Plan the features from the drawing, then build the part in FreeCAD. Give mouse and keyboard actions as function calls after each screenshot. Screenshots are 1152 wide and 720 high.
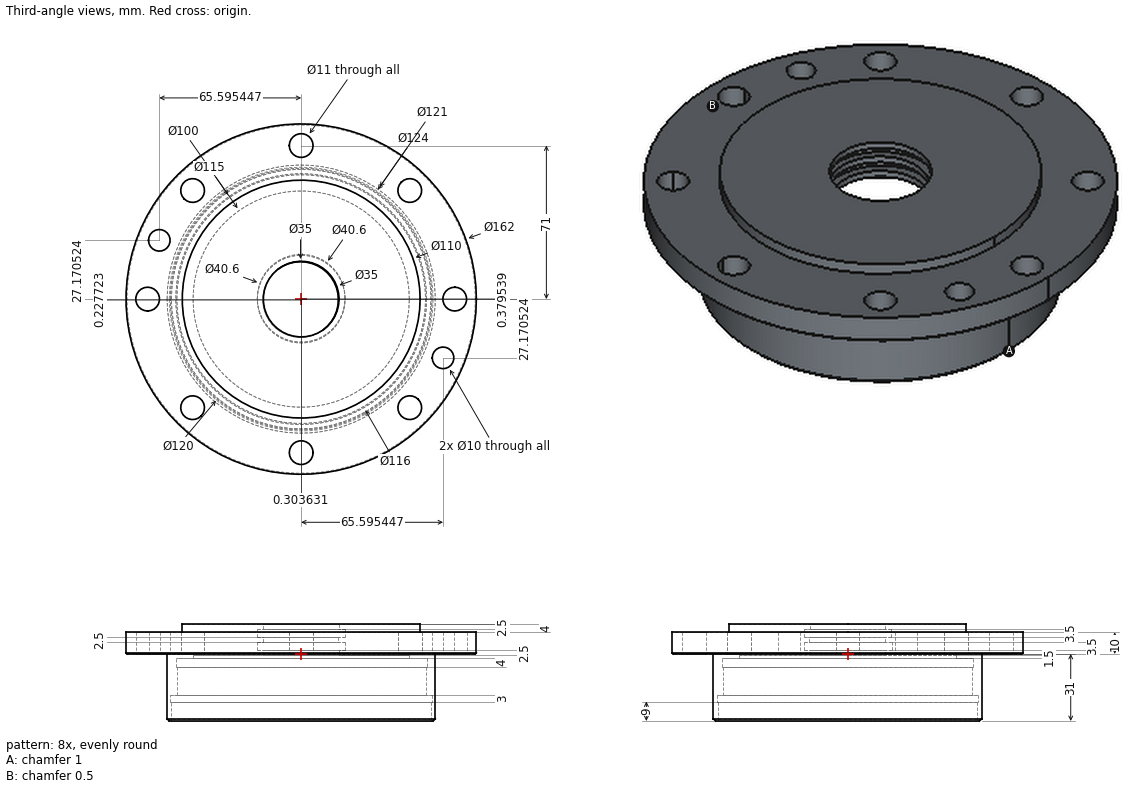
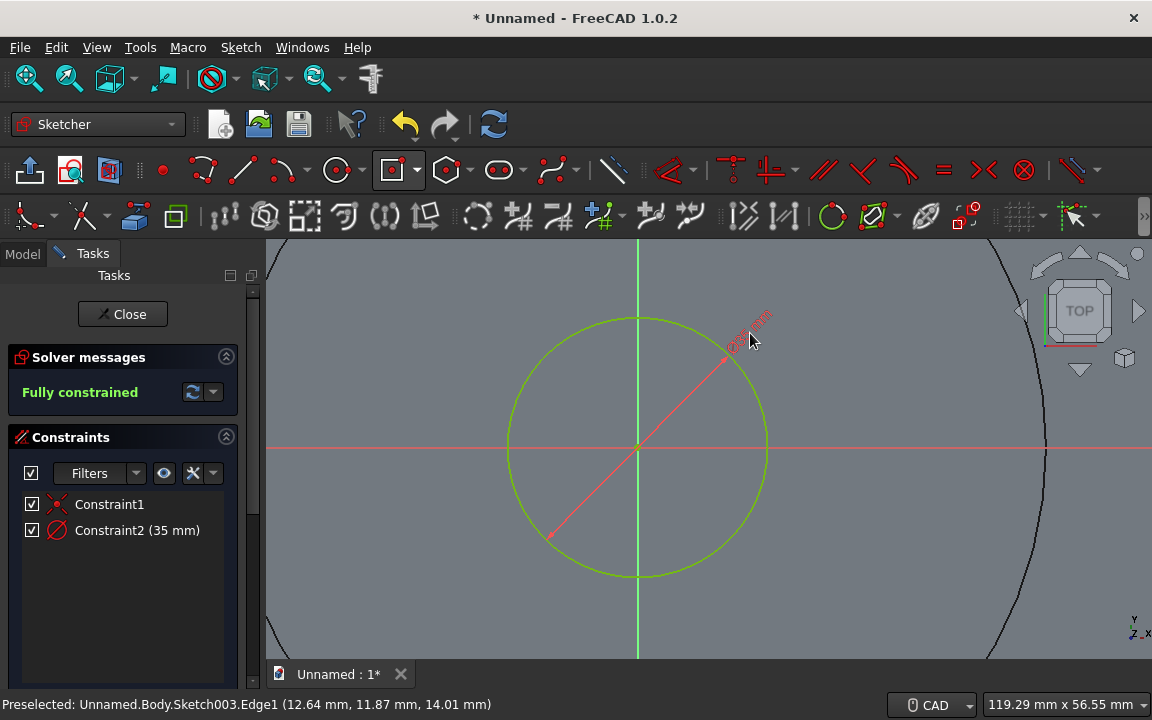
click(123, 314)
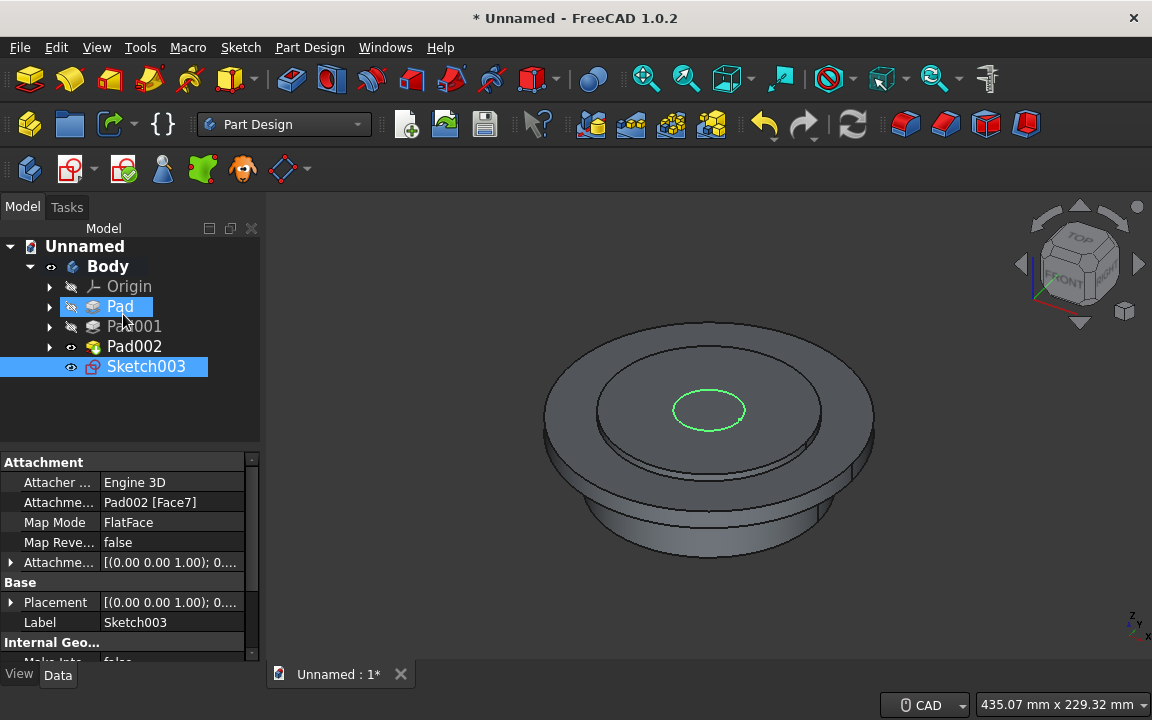
click(292, 80)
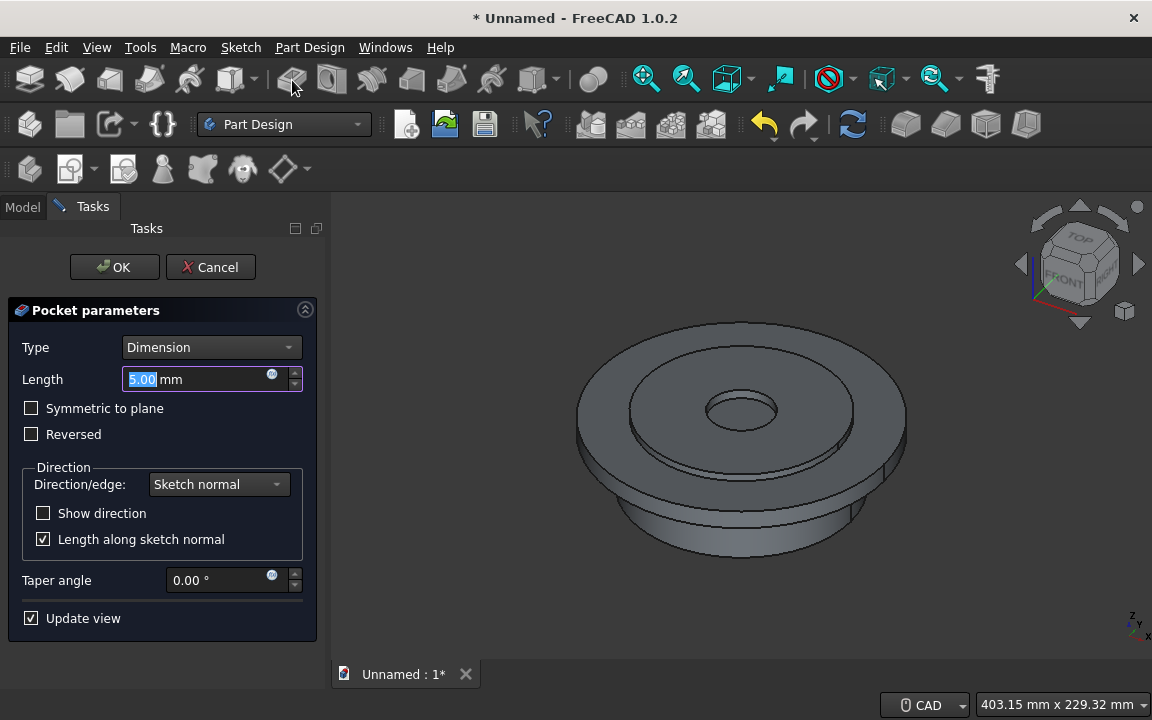
text(2.5)
key(Tab)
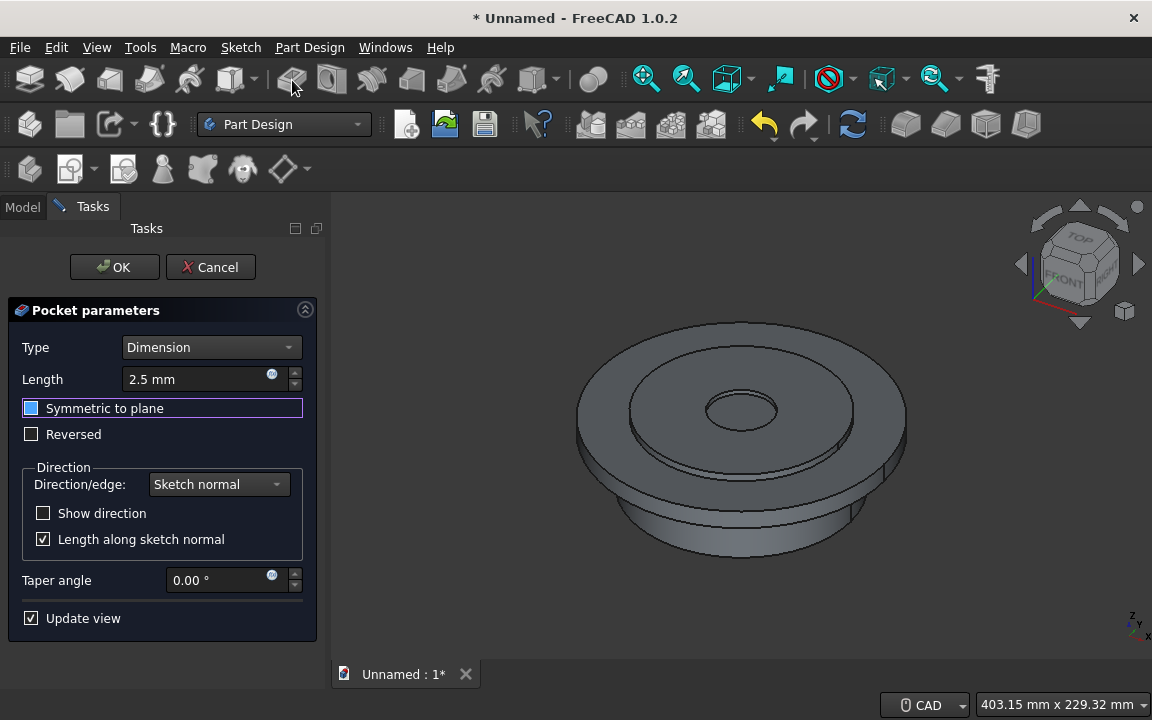
click(115, 267)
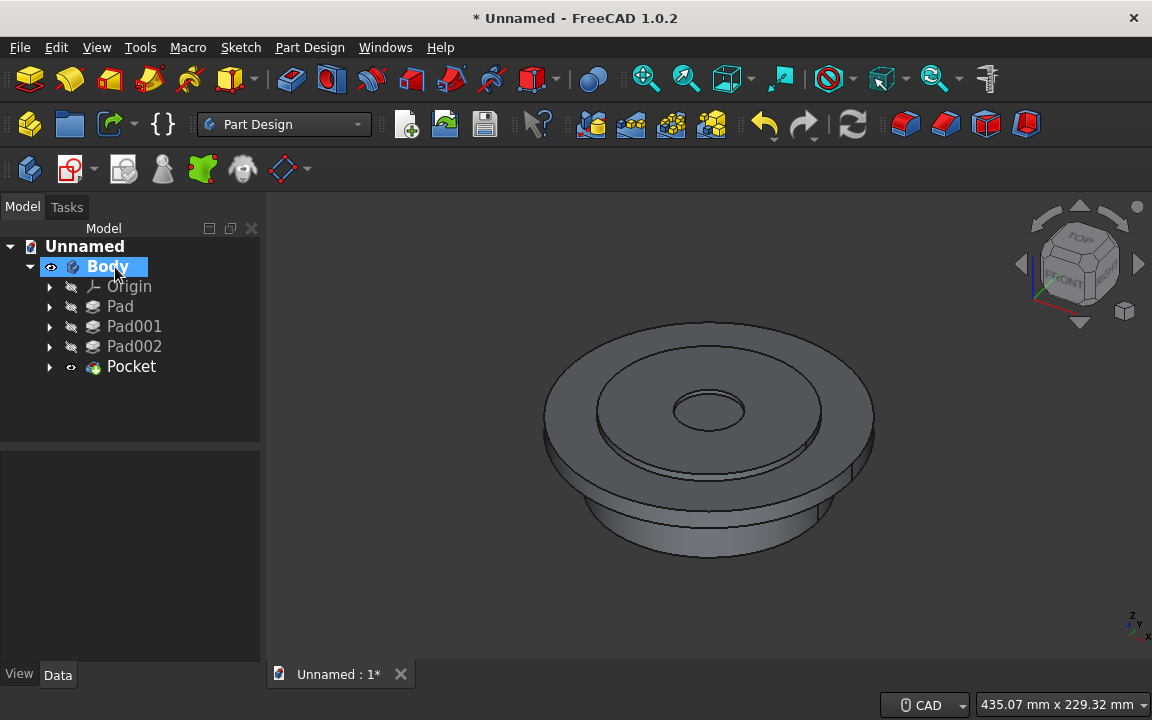
click(709, 413)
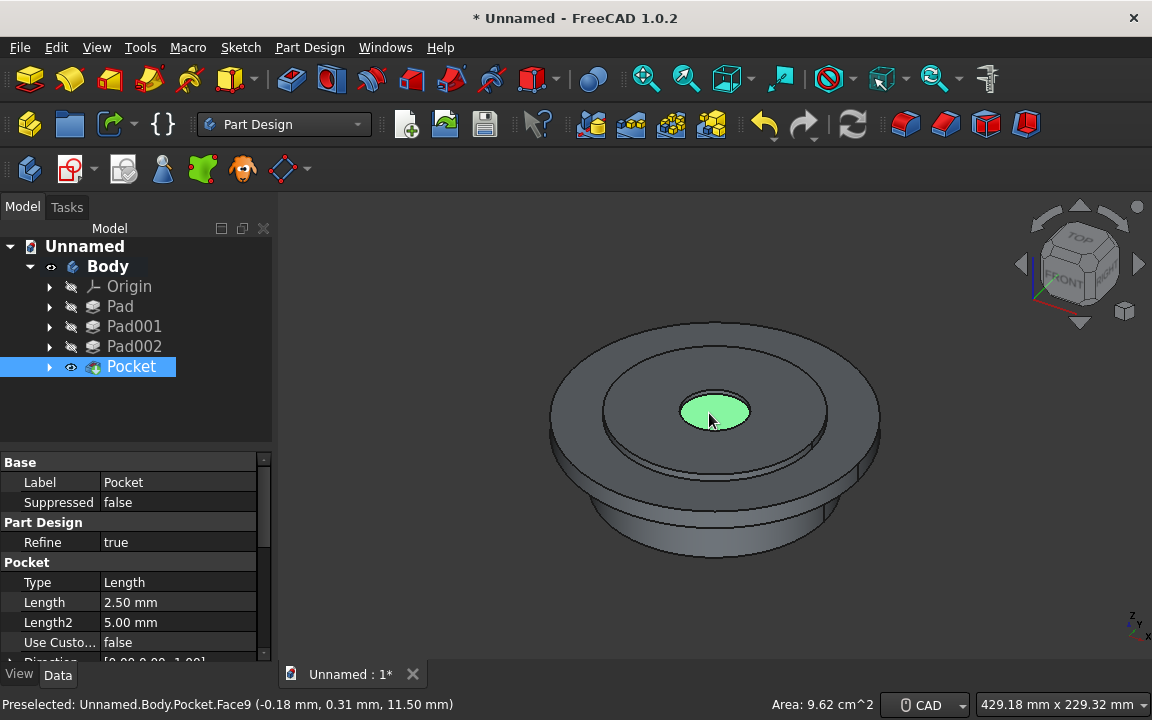
click(70, 170)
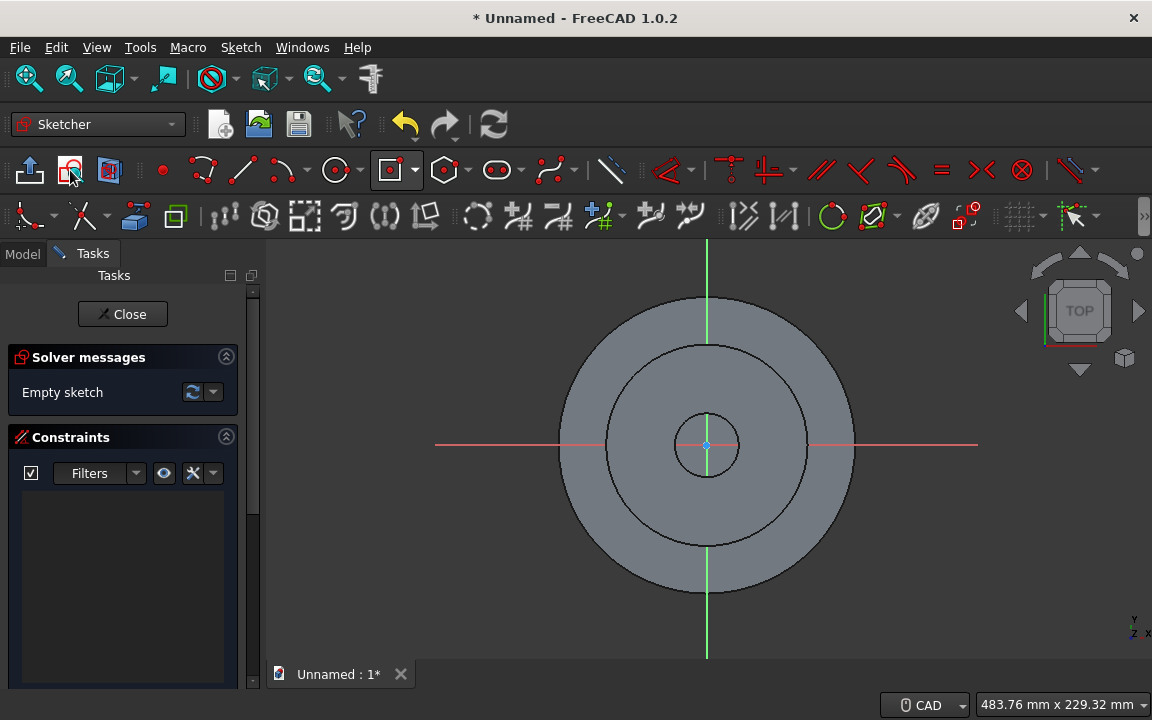
scroll(735, 444, up, 6)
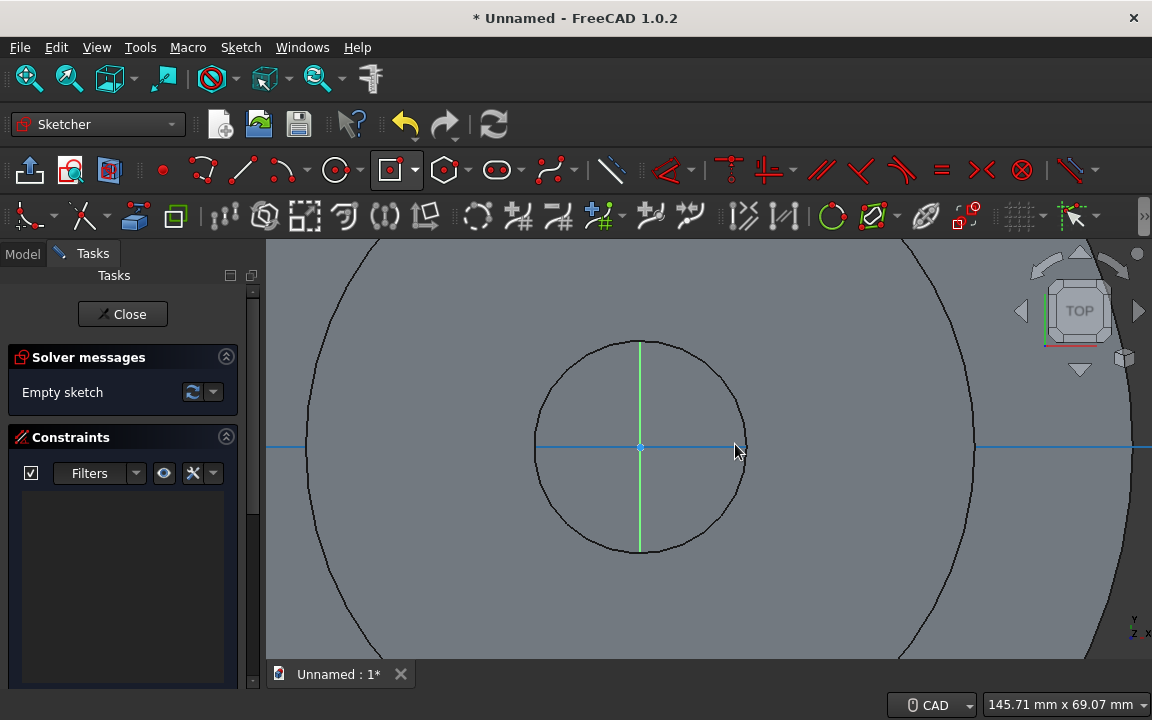
key(g)
key(c)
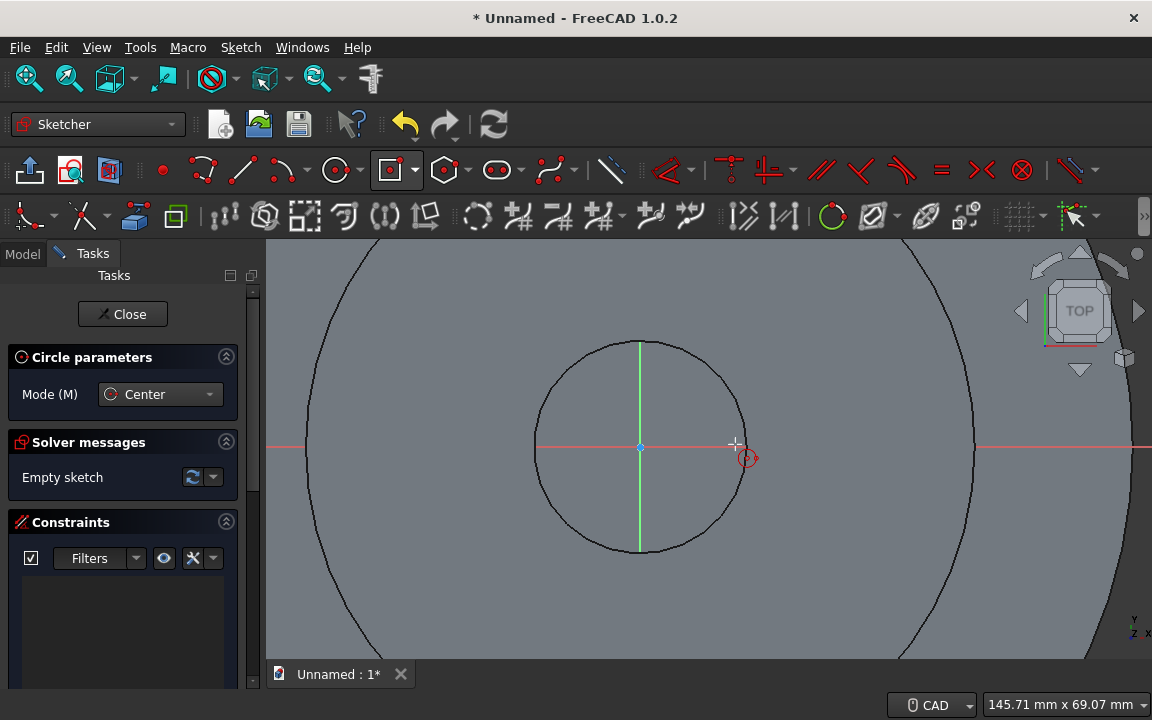
click(640, 447)
click(728, 360)
key(Escape)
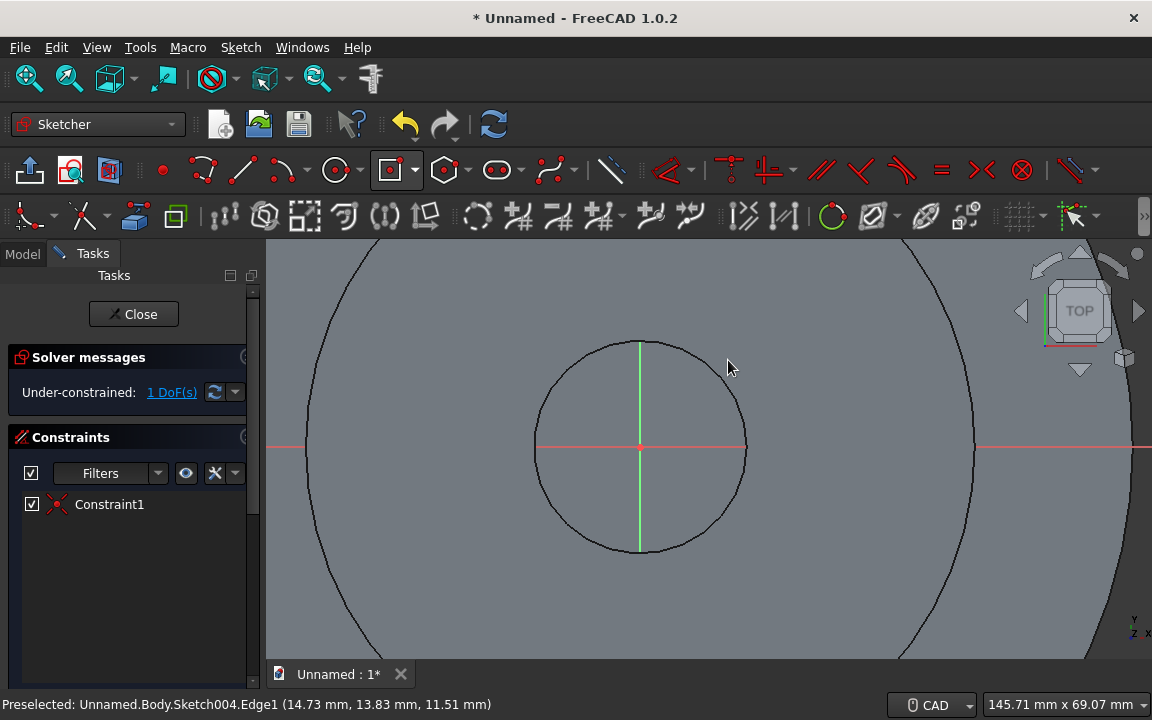
key(d)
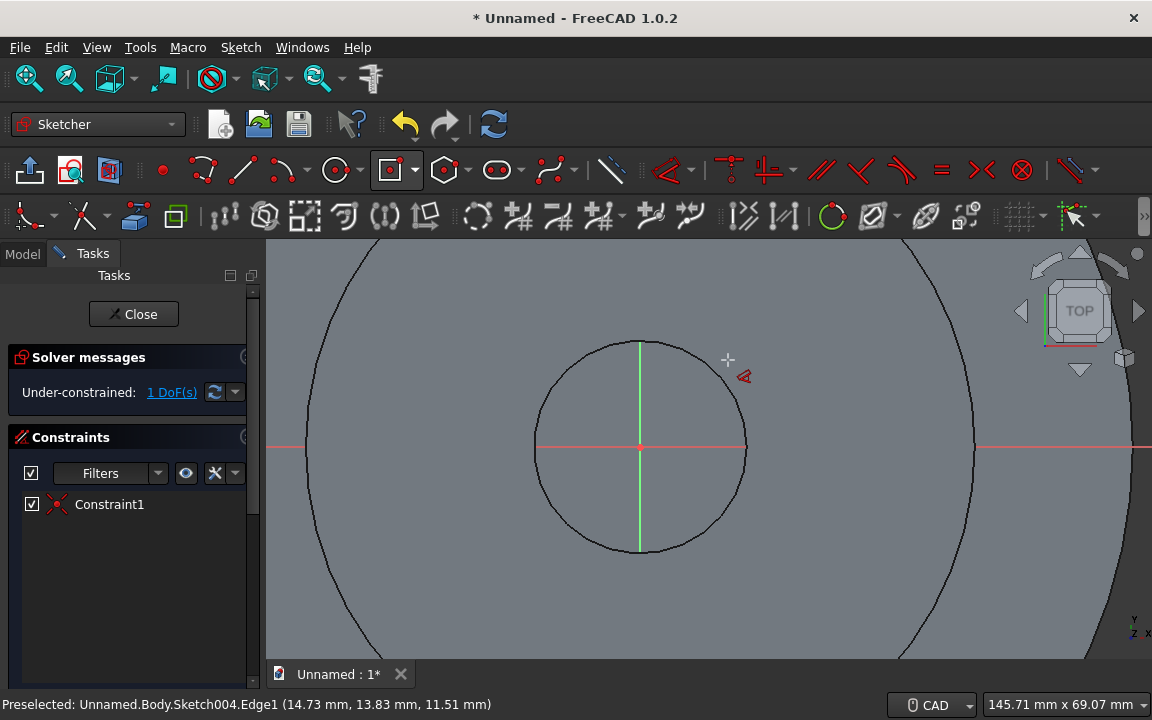
click(727, 360)
click(750, 337)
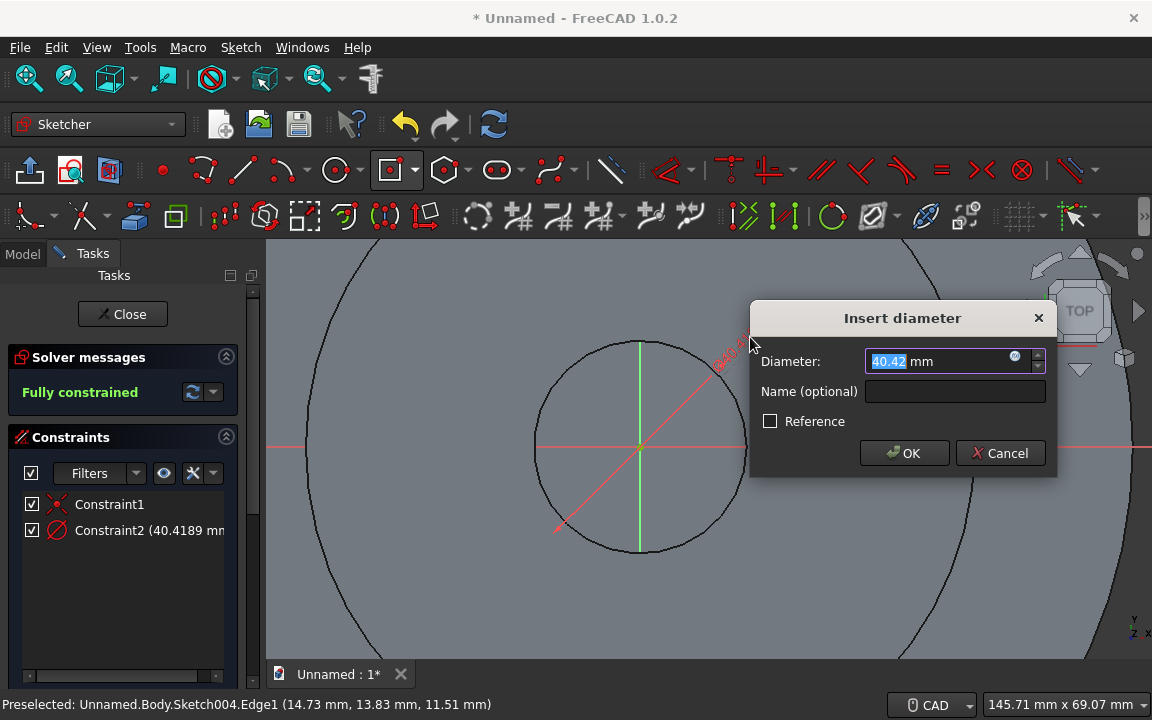
text(40.6)
key(Return)
key(Escape)